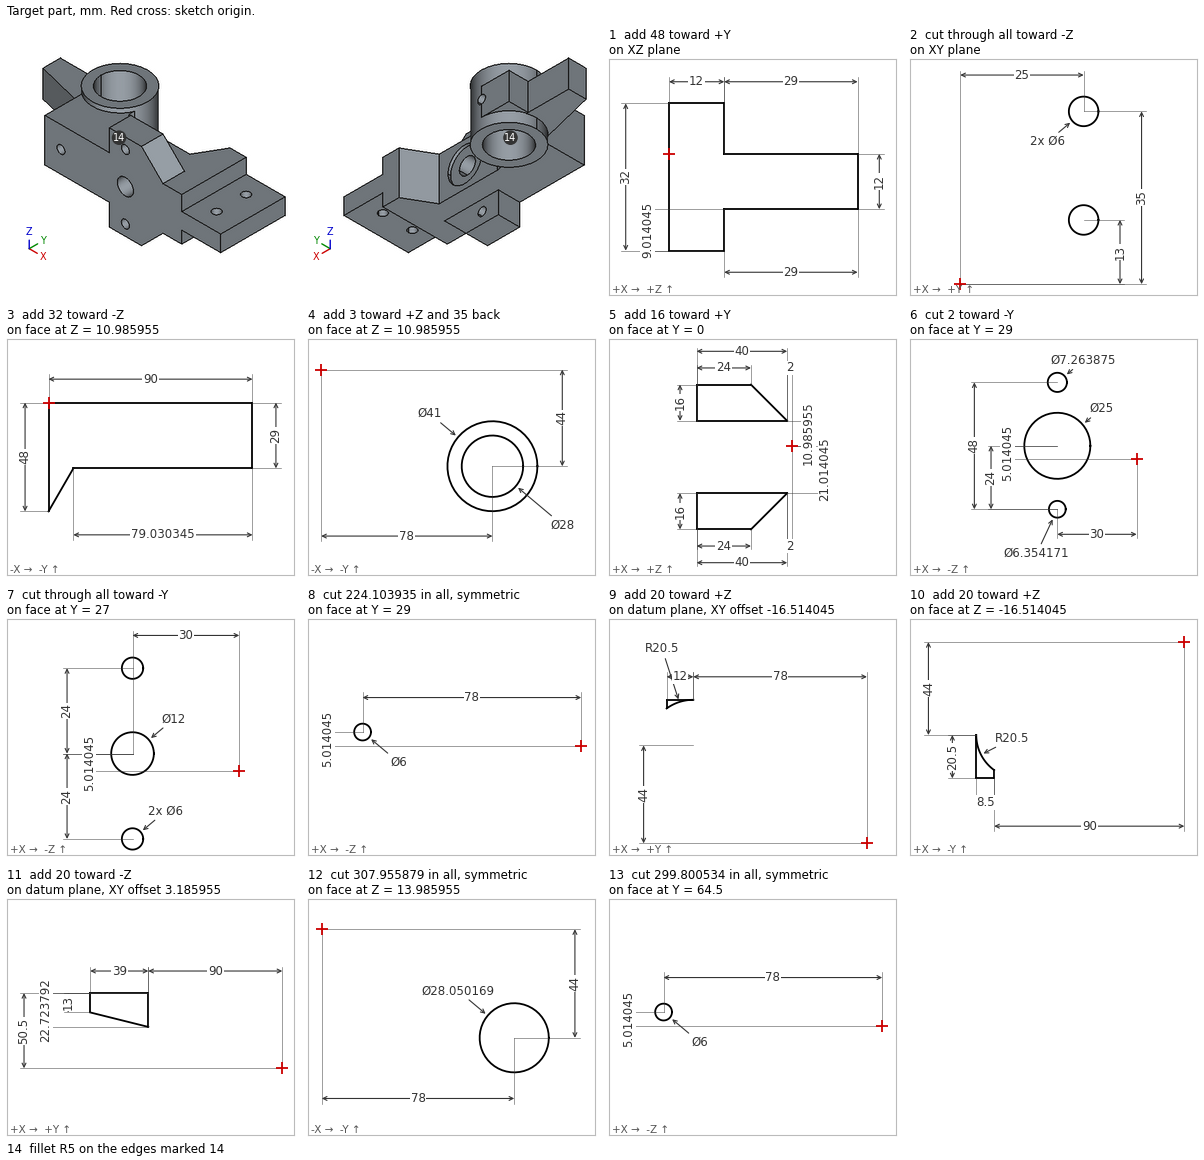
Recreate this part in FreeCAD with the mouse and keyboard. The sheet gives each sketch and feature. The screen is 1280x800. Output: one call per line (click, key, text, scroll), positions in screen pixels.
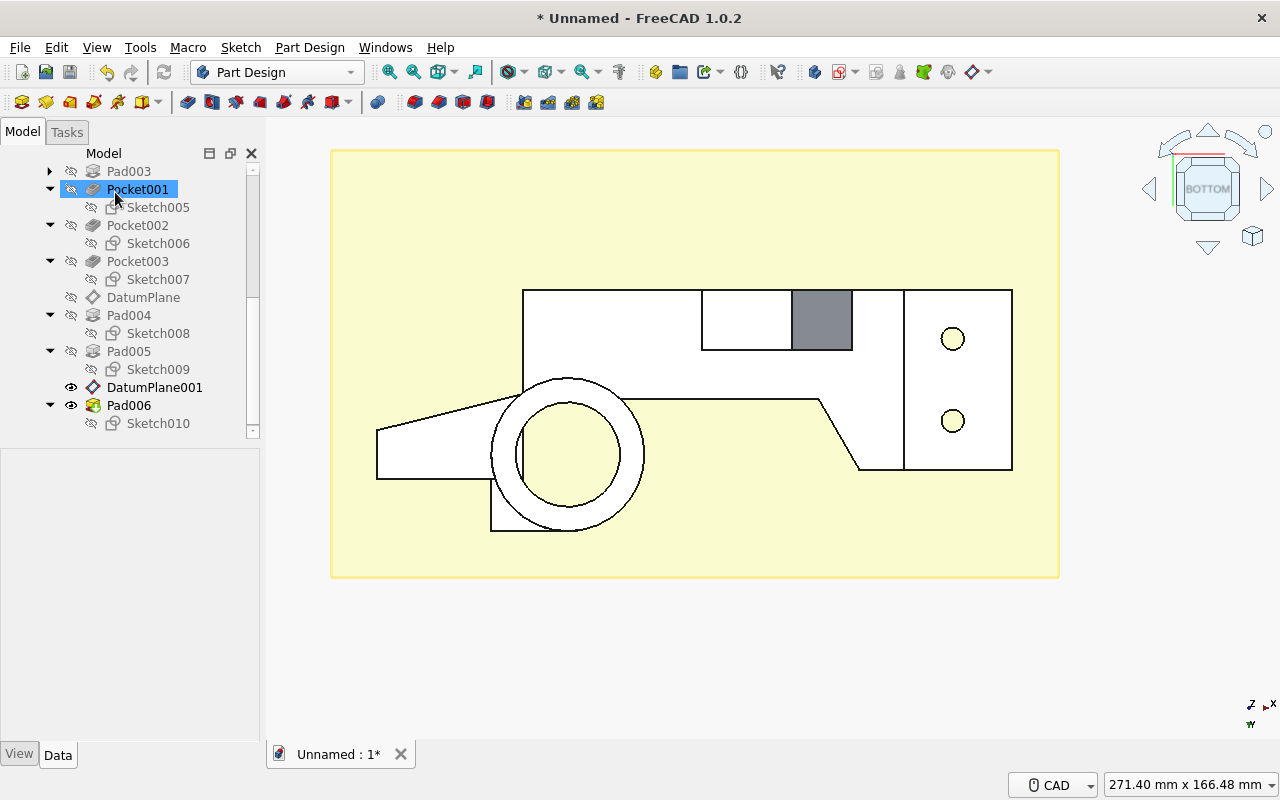
click(116, 387)
key(space)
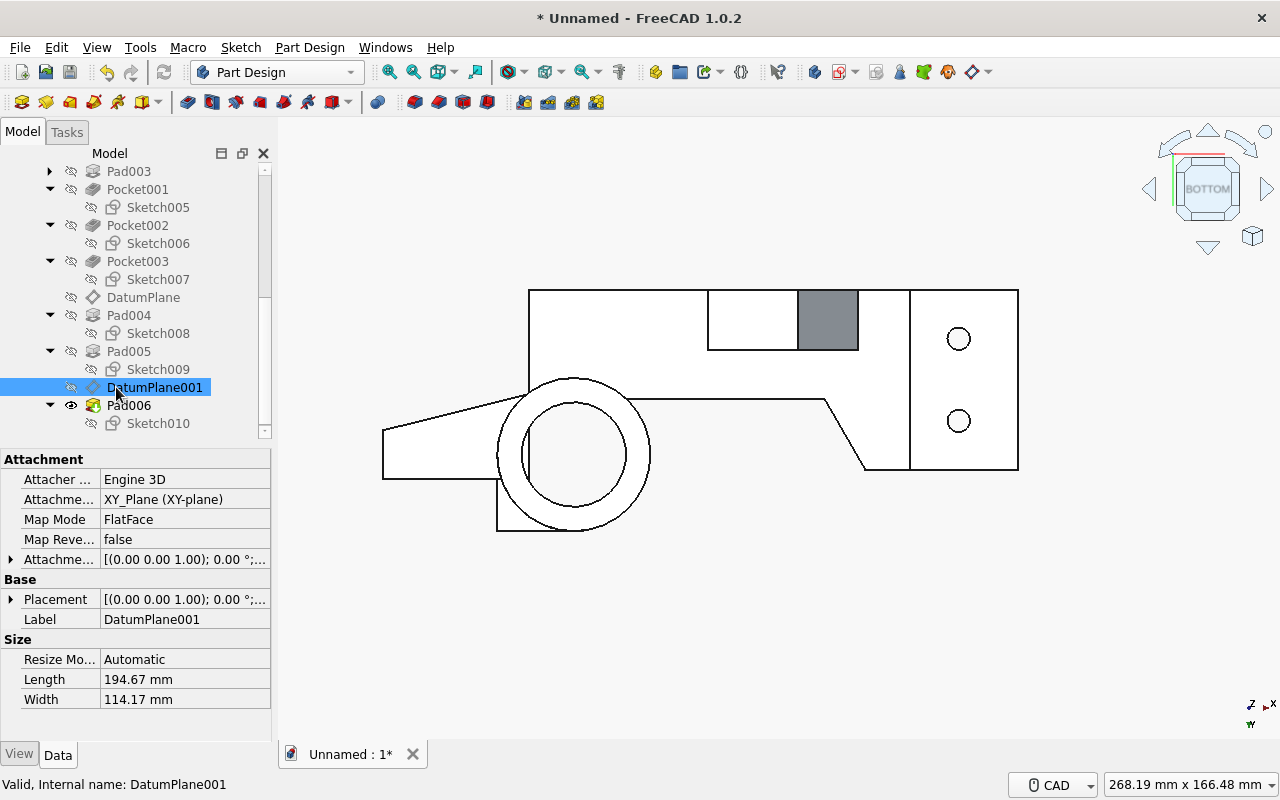
key(0)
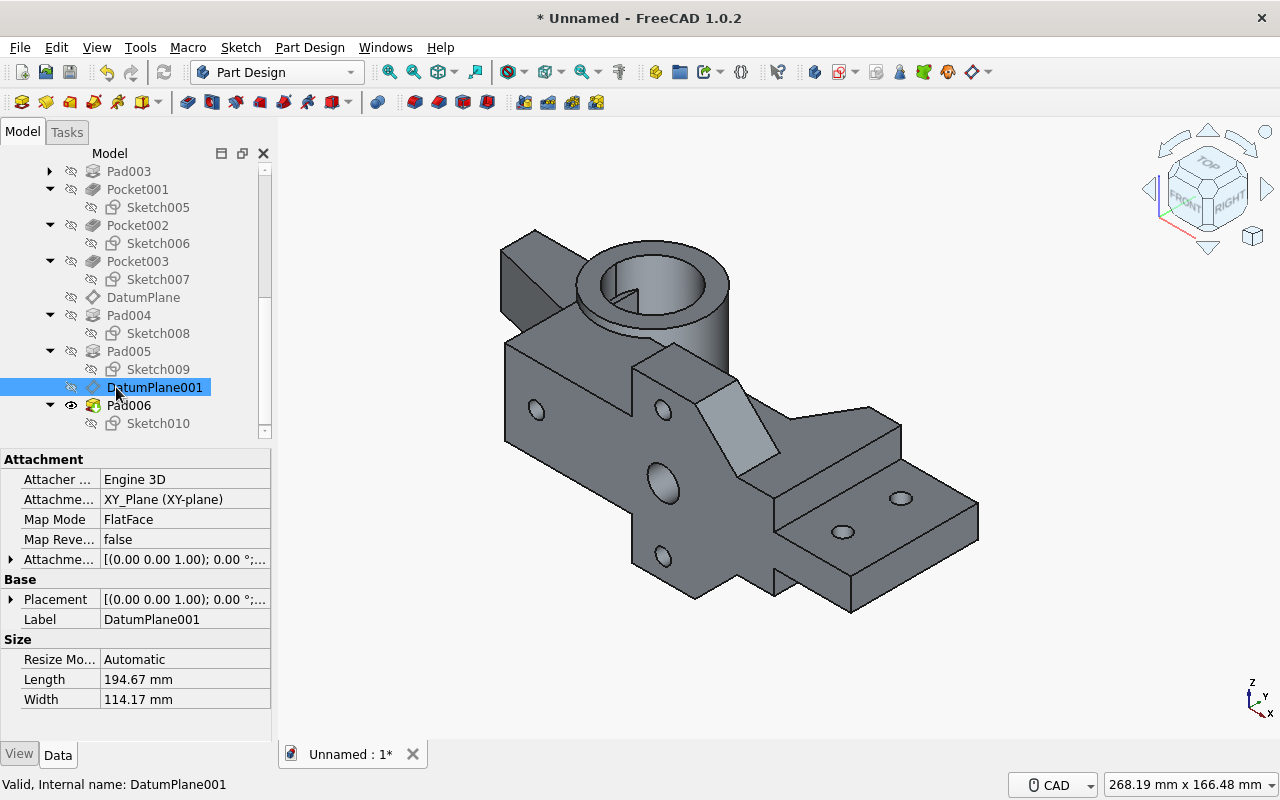
click(699, 257)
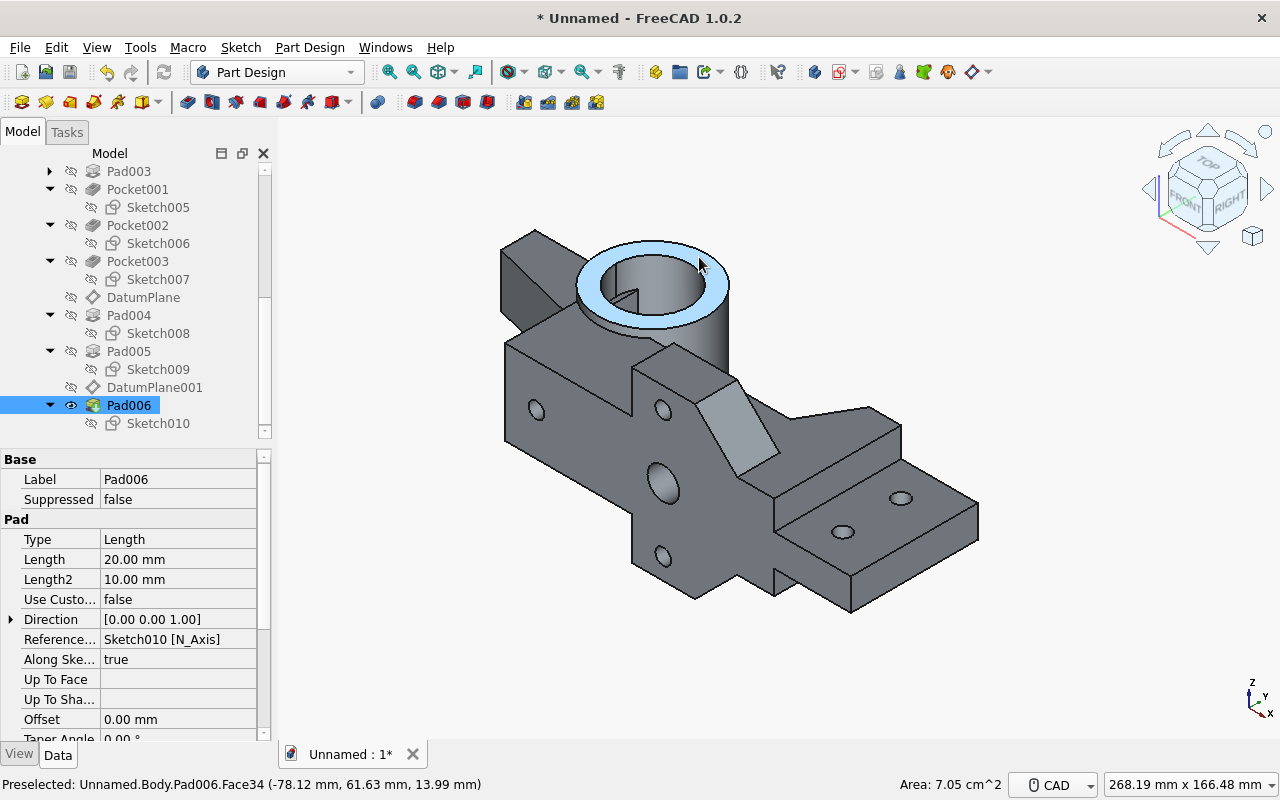
click(840, 72)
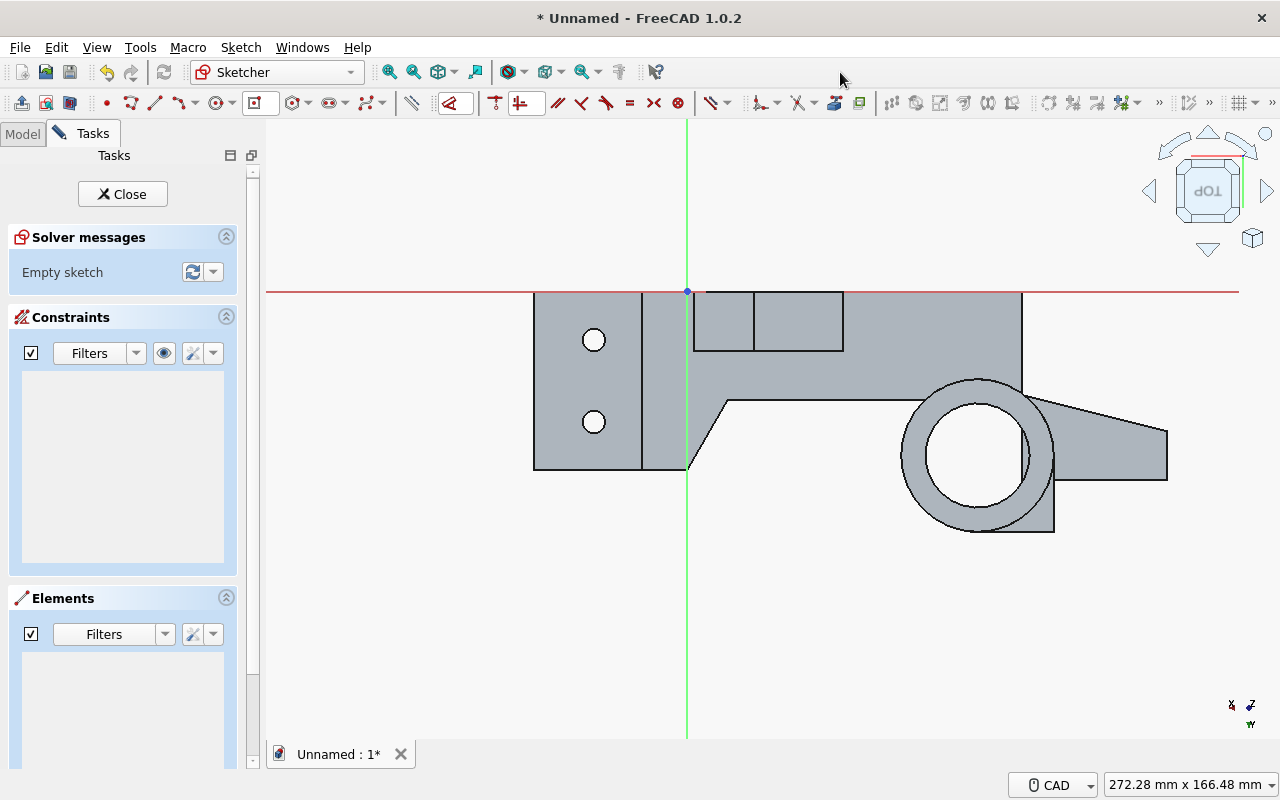
click(70, 104)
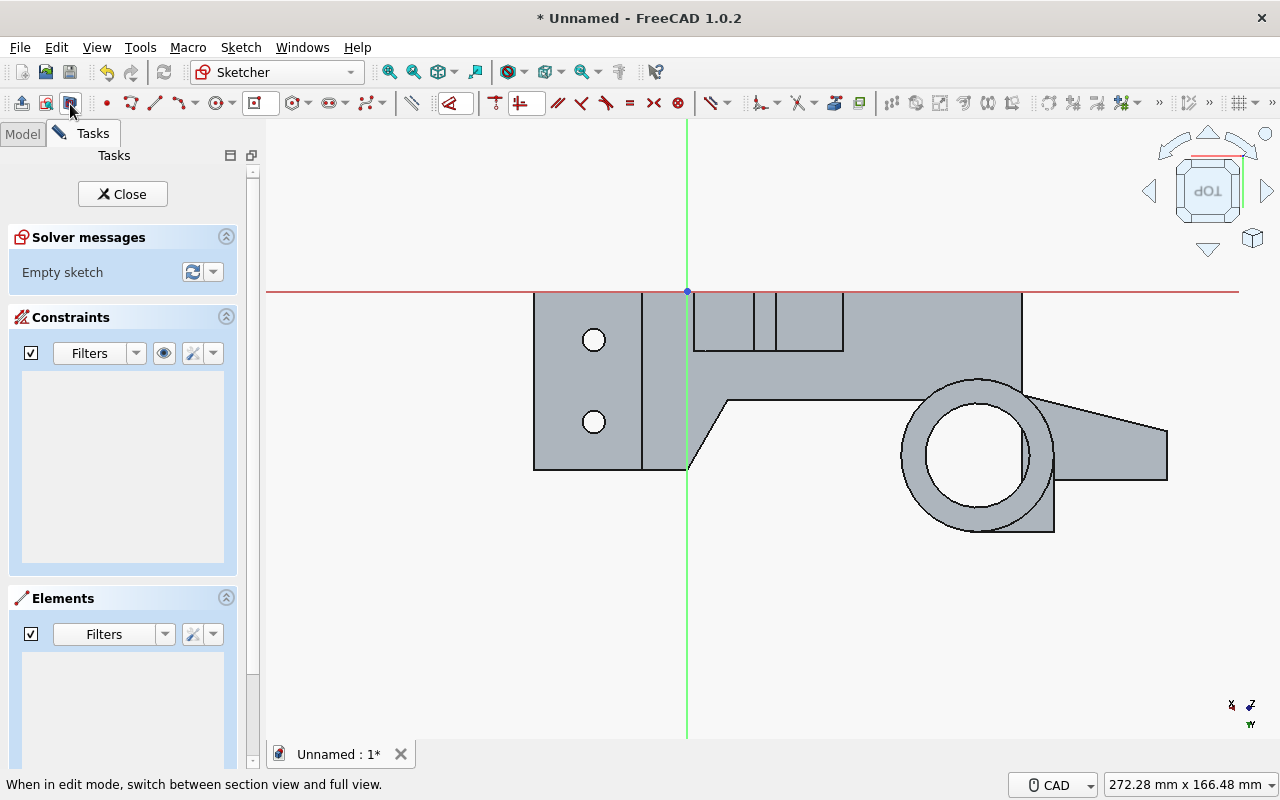
scroll(1067, 464, up, 7)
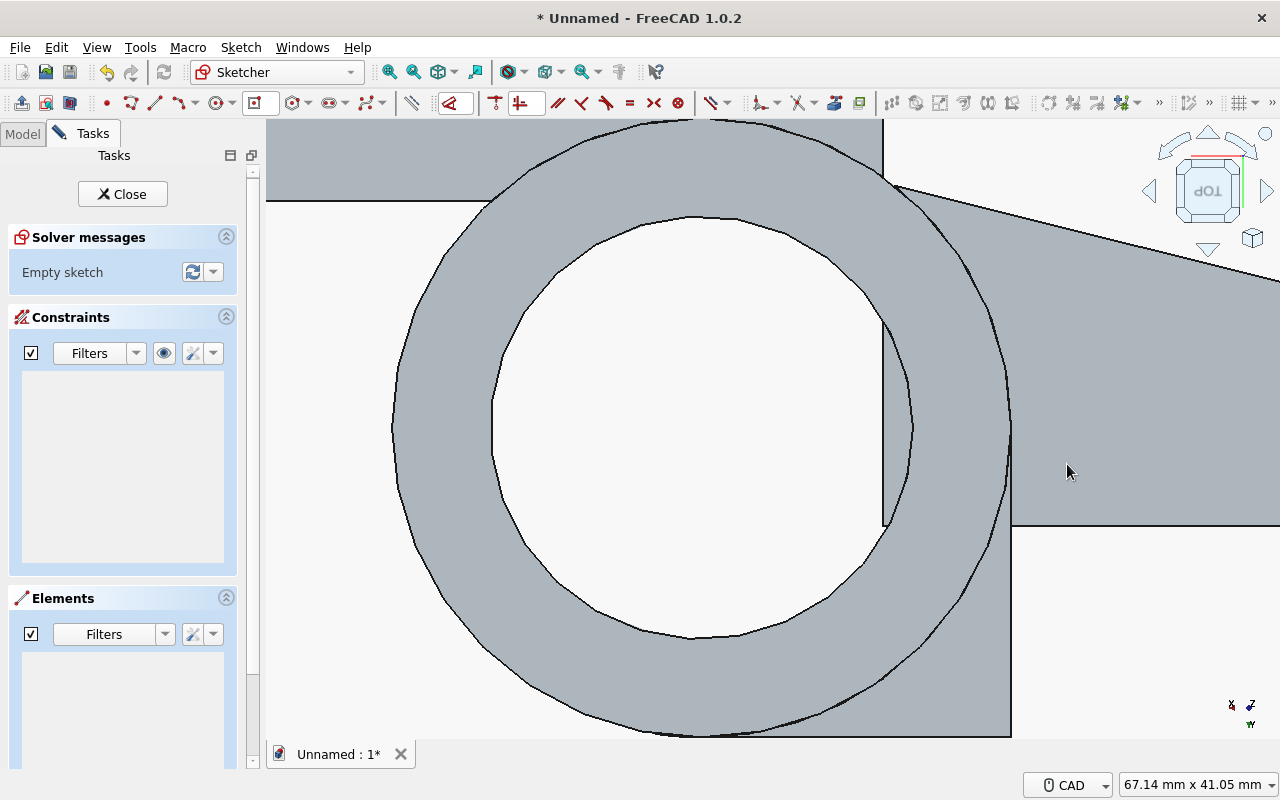
key(g)
key(c)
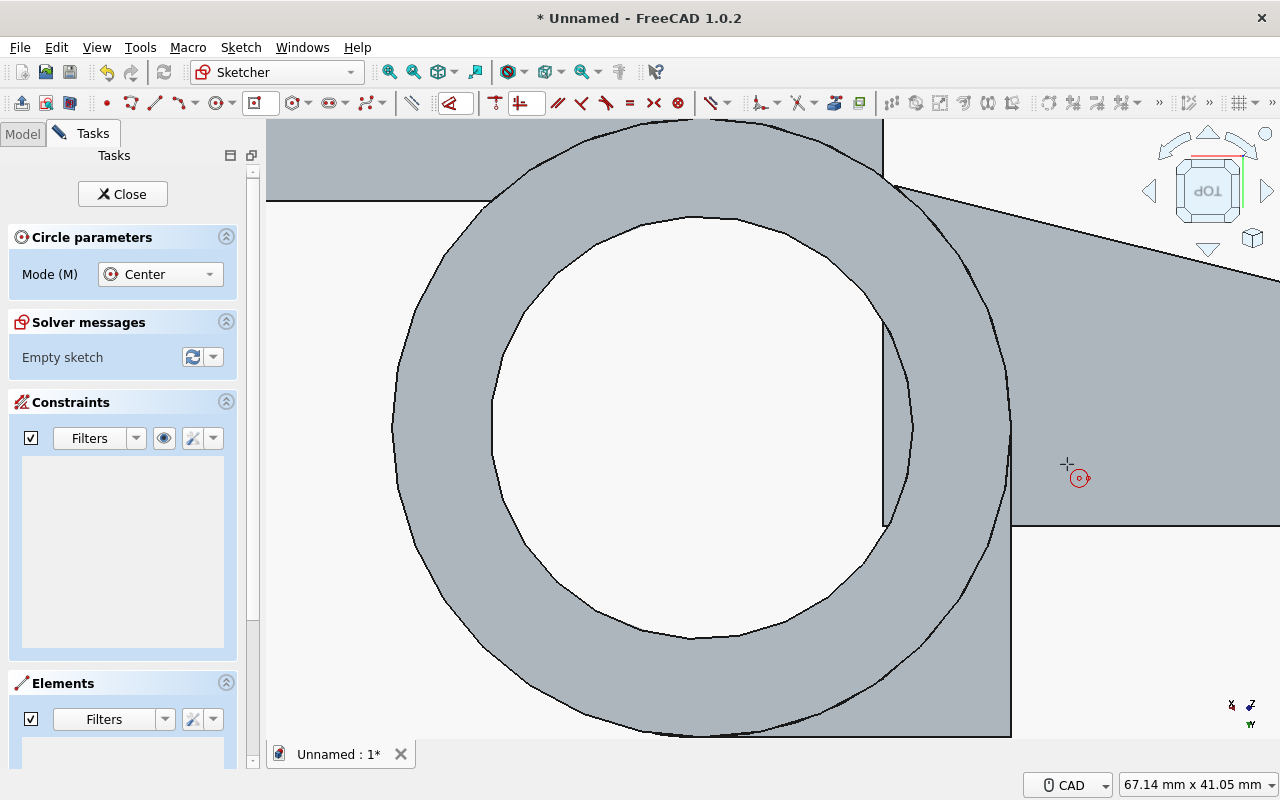
click(702, 428)
move(851, 278)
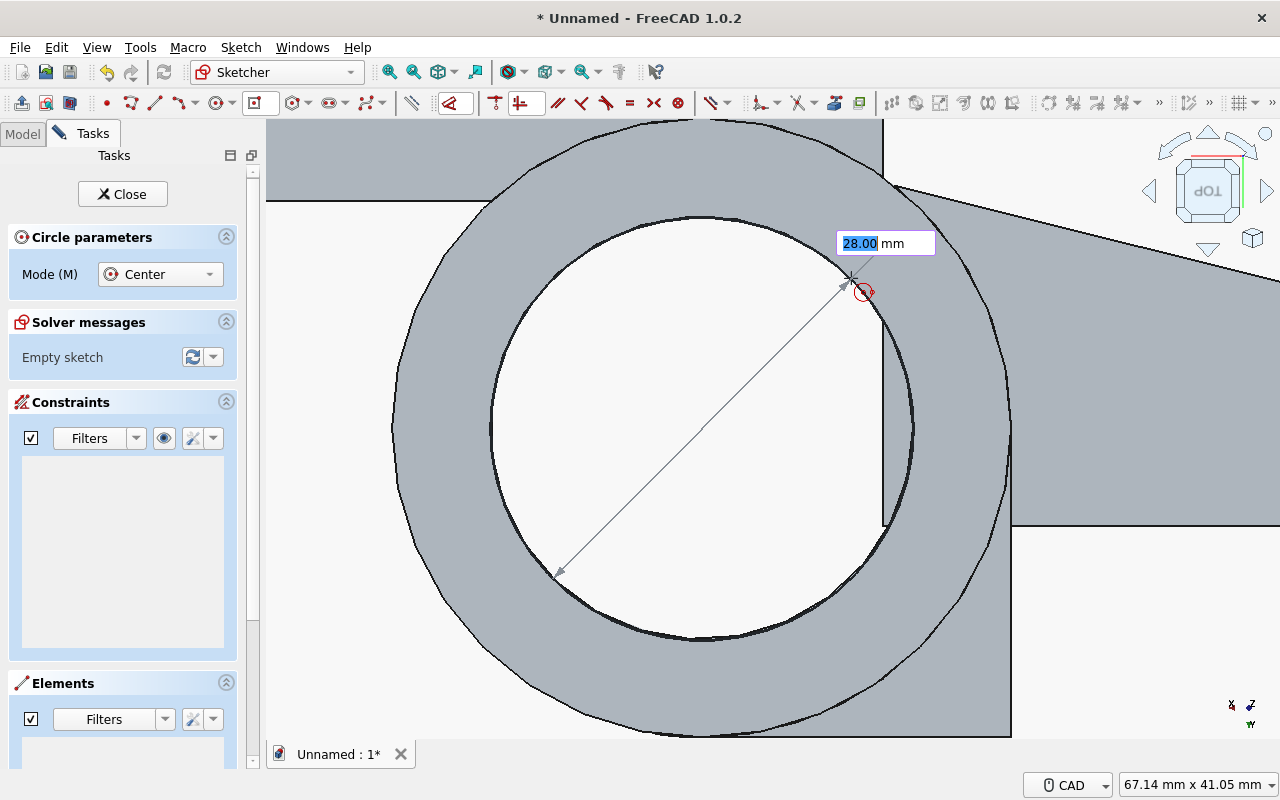
text(28.050169)
key(Return)
key(Escape)